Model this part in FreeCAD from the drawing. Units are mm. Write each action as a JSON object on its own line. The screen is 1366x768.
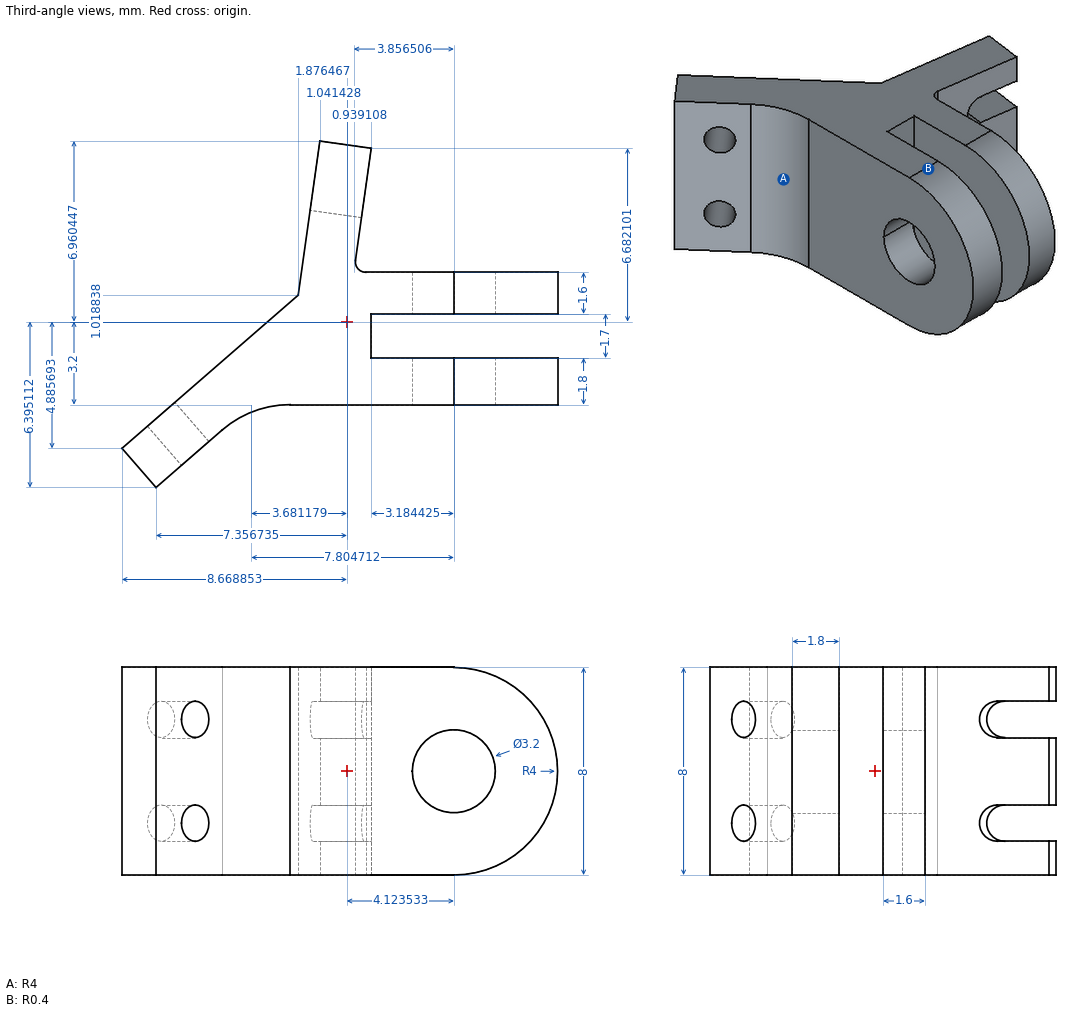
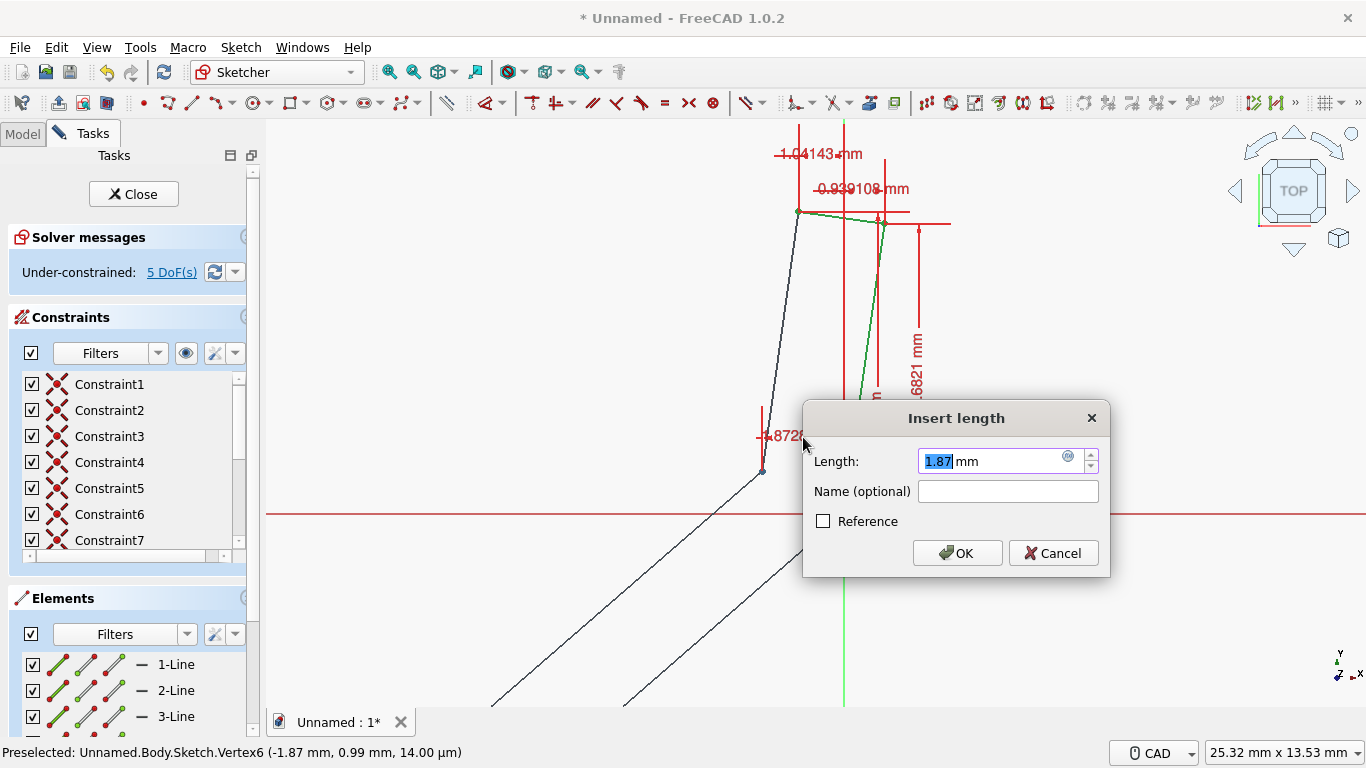
{"action": "type", "text": "1.876467"}
{"action": "key", "text": "Return"}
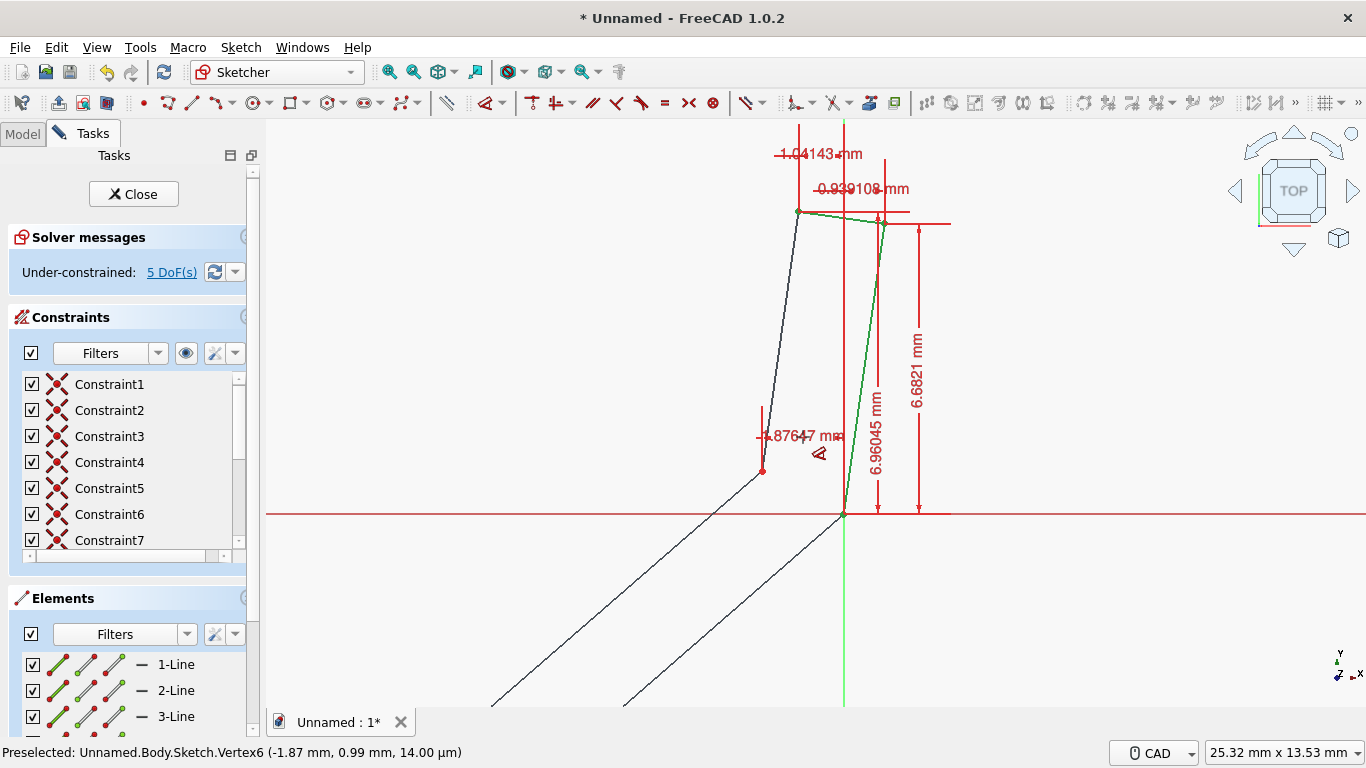
{"action": "left_click", "coordinate": [762, 471]}
{"action": "left_click", "coordinate": [878, 493]}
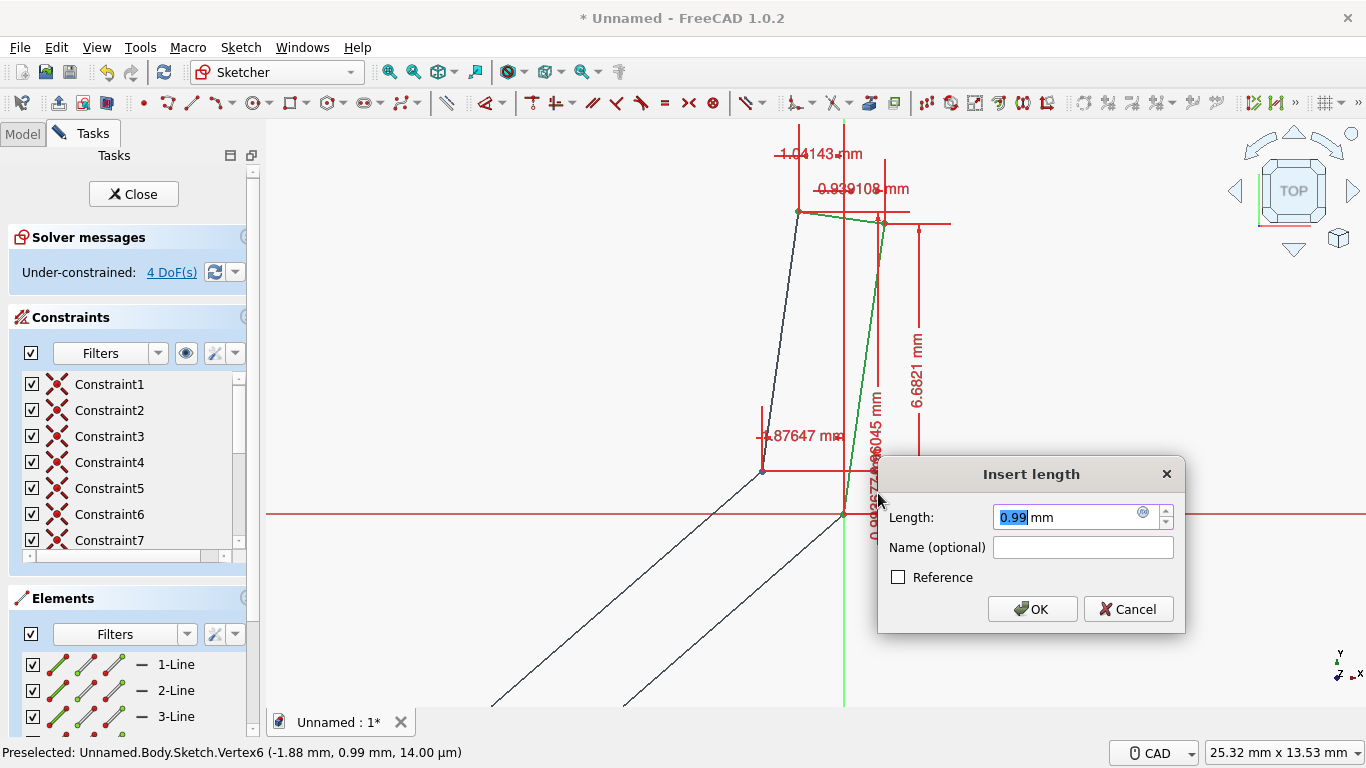
{"action": "type", "text": "1.018838"}
{"action": "key", "text": "Return"}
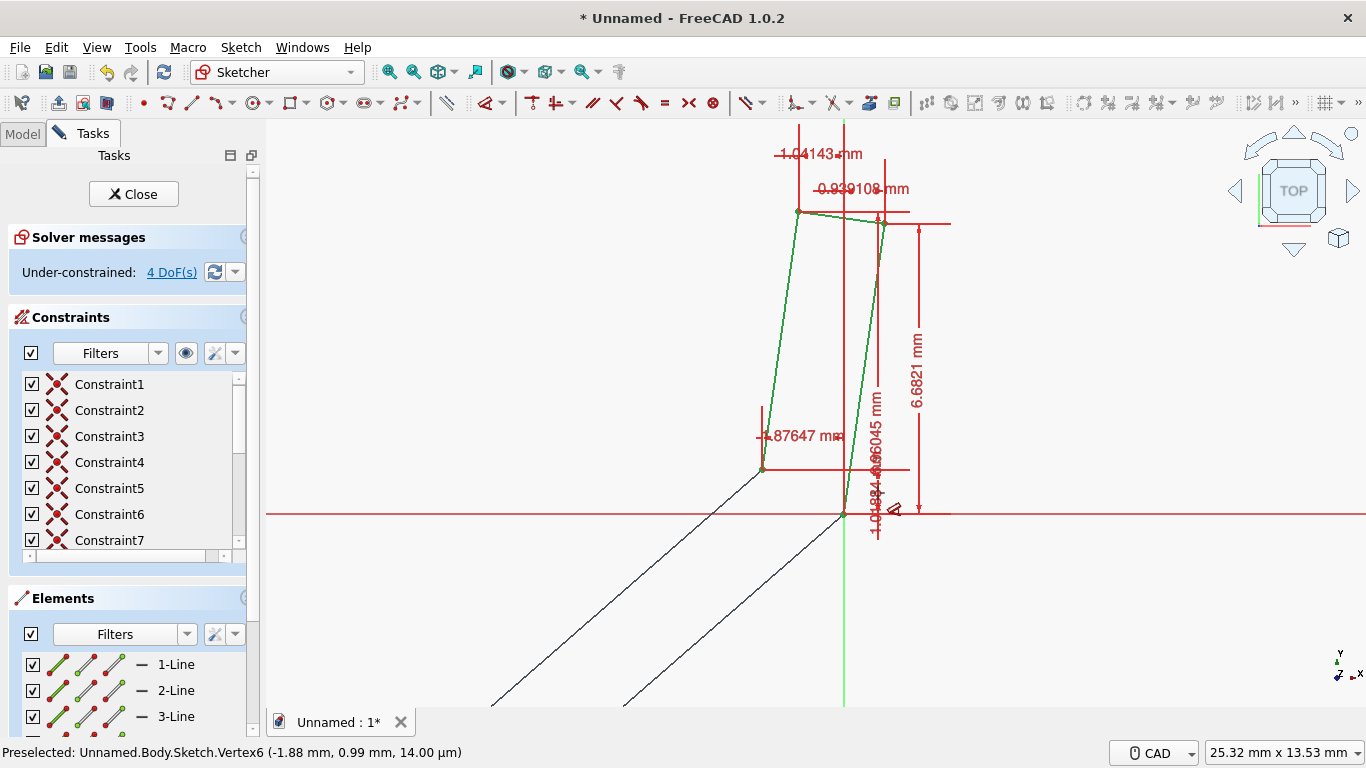
{"action": "scroll", "coordinate": [893, 232], "scroll_direction": "down", "scroll_amount": 2}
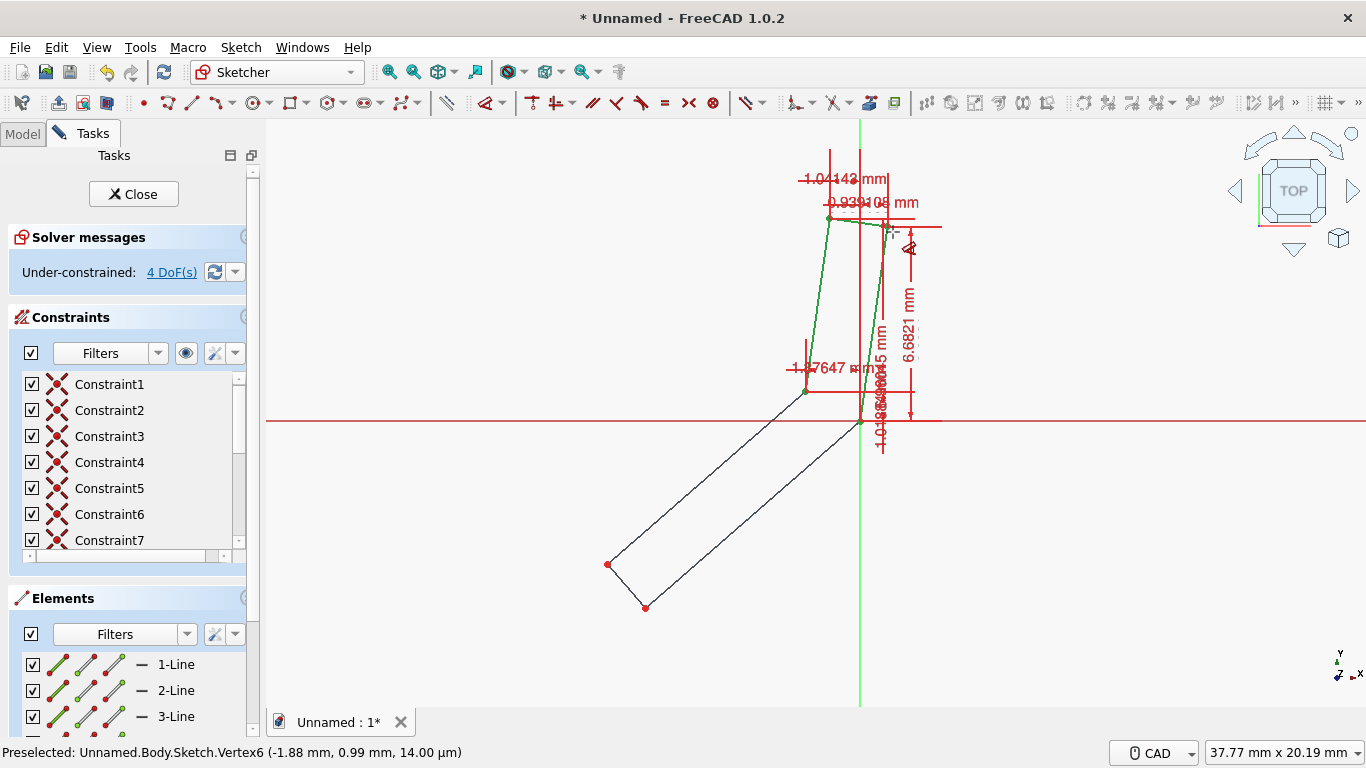
{"action": "left_click", "coordinate": [608, 564]}
{"action": "left_click", "coordinate": [734, 598]}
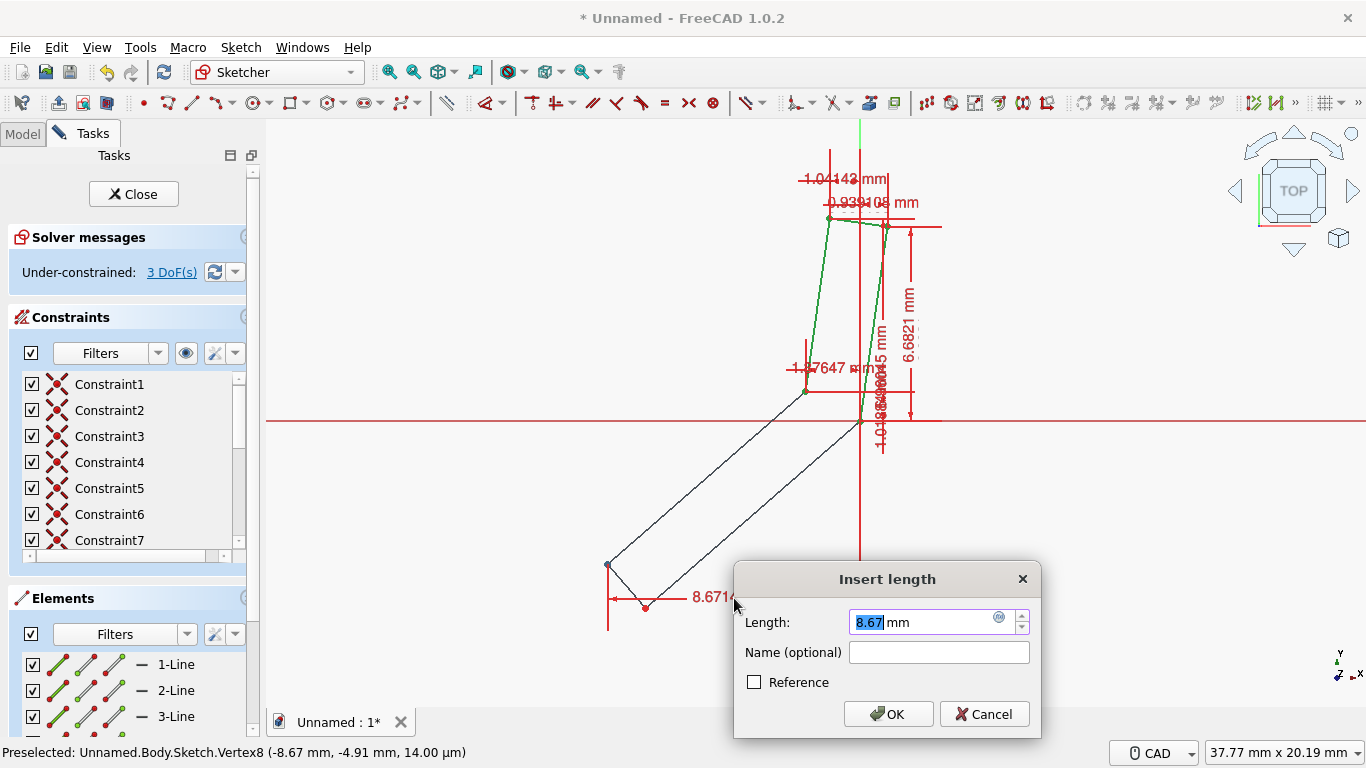
{"action": "type", "text": "8.668853"}
{"action": "key", "text": "Return"}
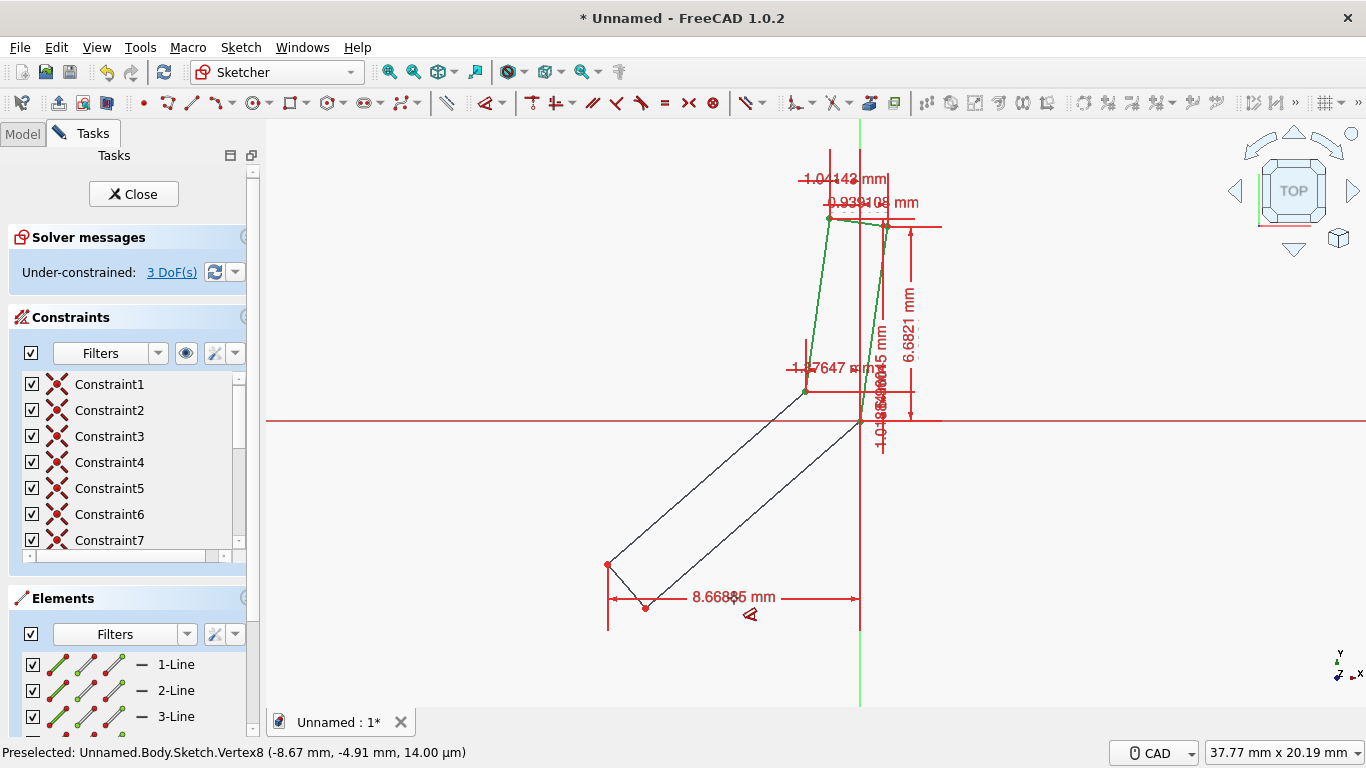
{"action": "left_click", "coordinate": [608, 564]}
{"action": "left_click", "coordinate": [574, 493]}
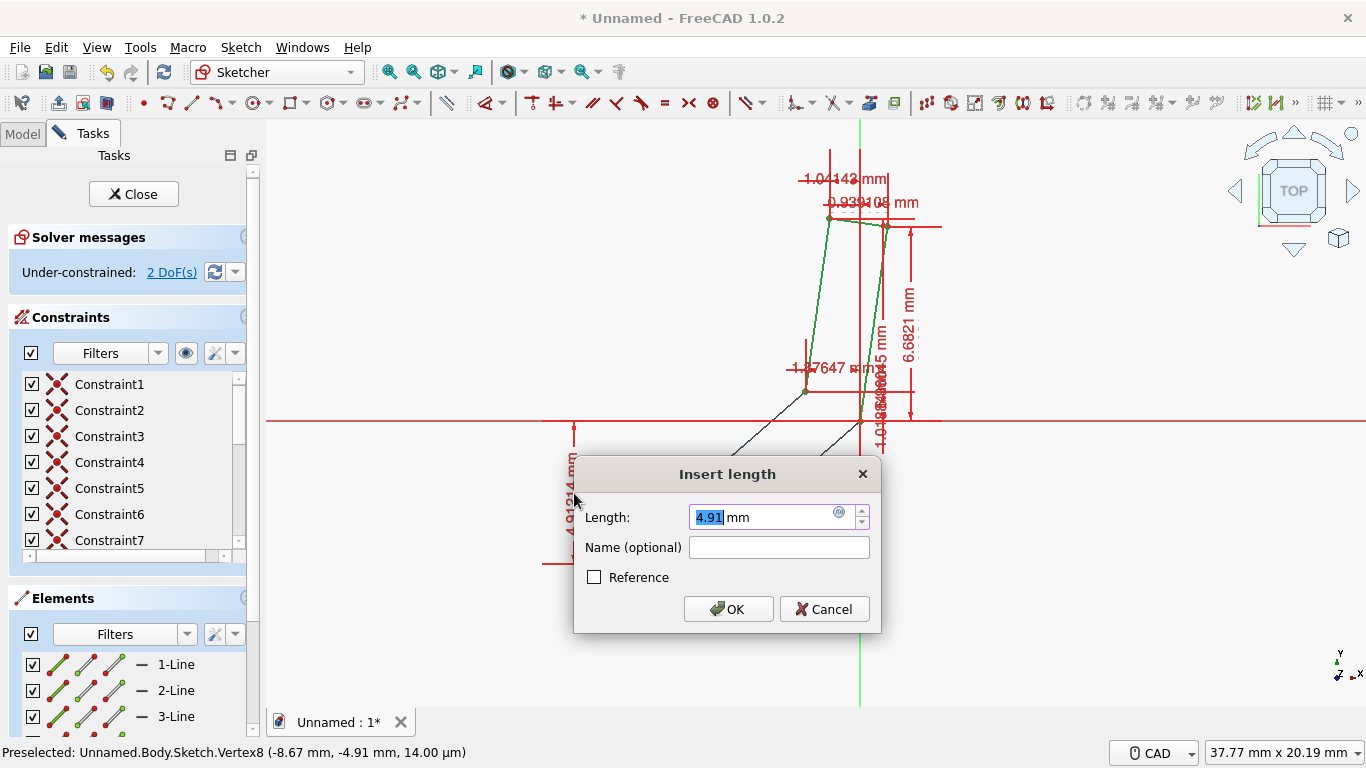
{"action": "type", "text": "4.885693"}
{"action": "key", "text": "Return"}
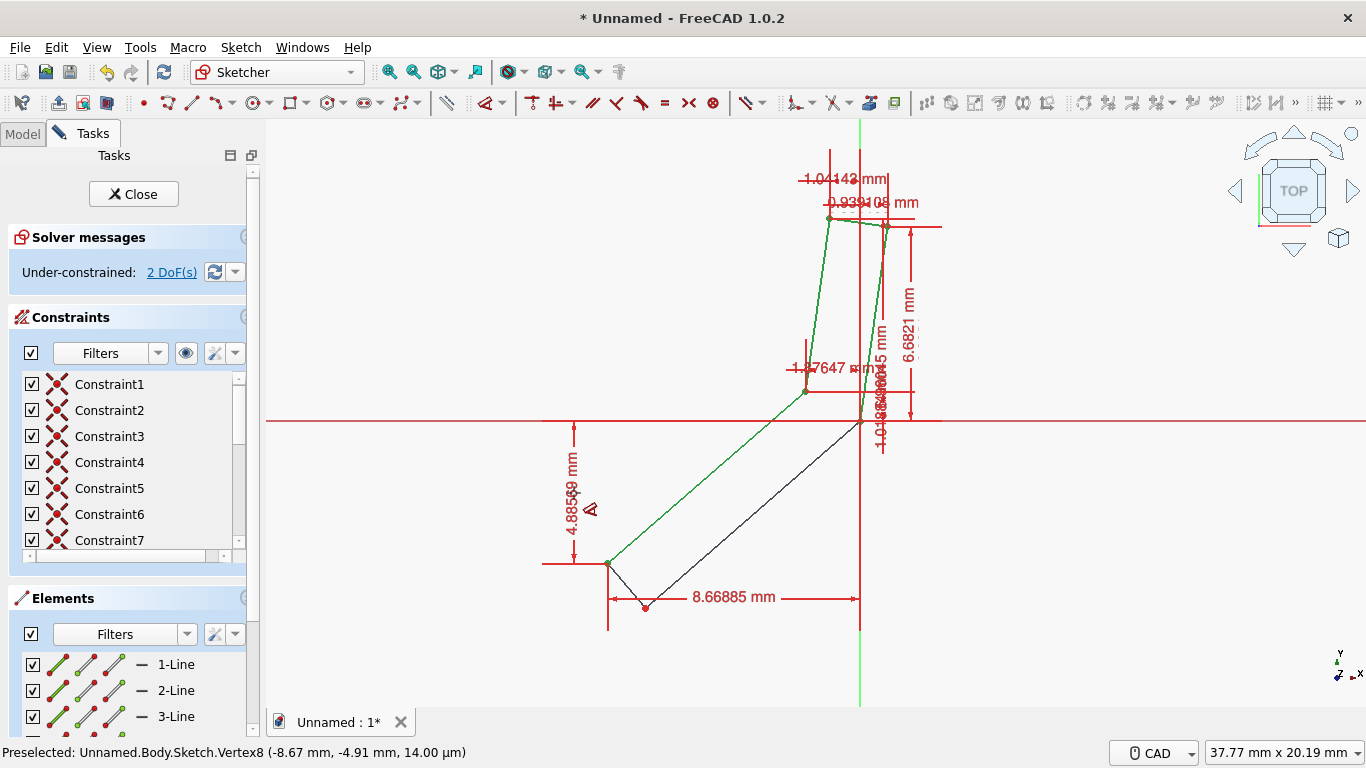
{"action": "left_click", "coordinate": [646, 608]}
{"action": "left_click", "coordinate": [753, 642]}